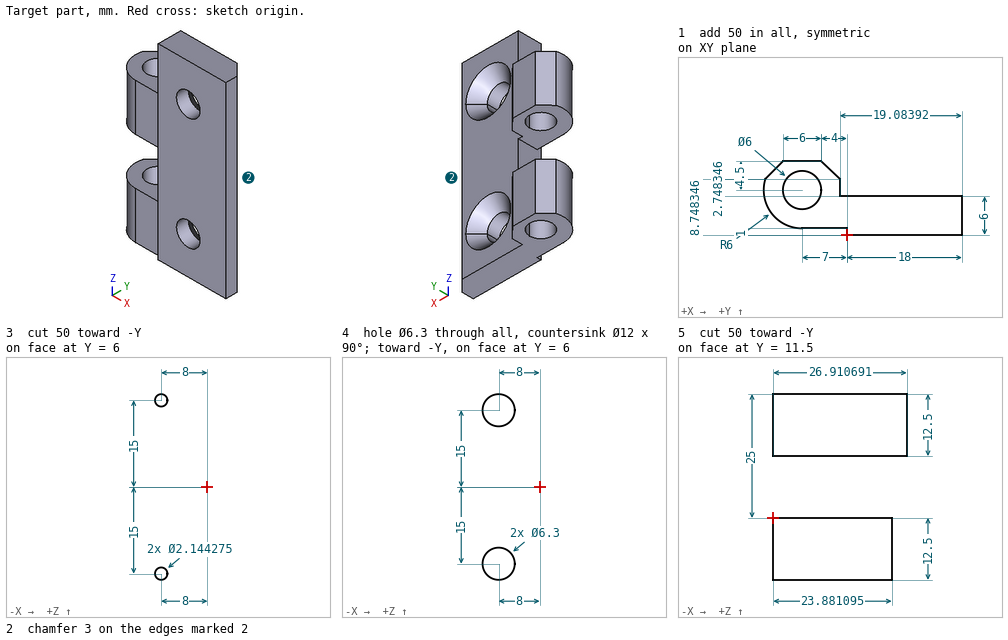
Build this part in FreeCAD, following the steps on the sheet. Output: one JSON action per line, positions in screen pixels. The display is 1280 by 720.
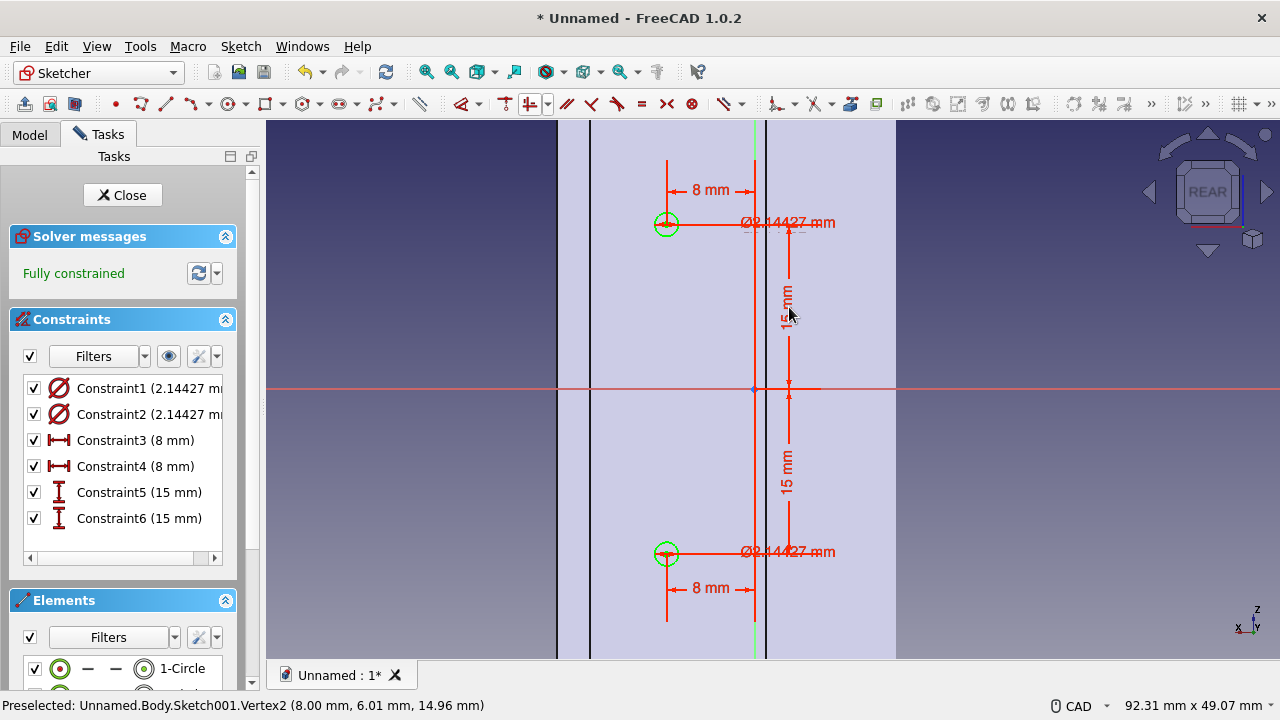
{"action": "left_click", "coordinate": [123, 195]}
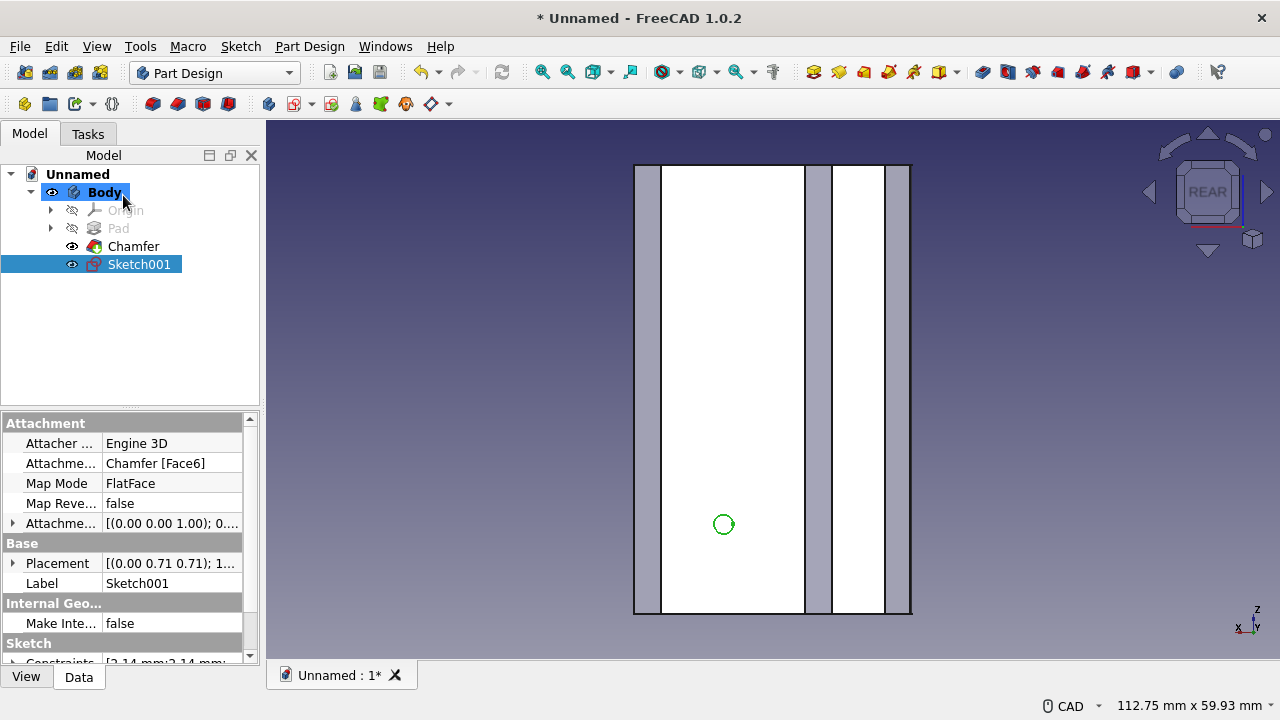
{"action": "left_click", "coordinate": [983, 72]}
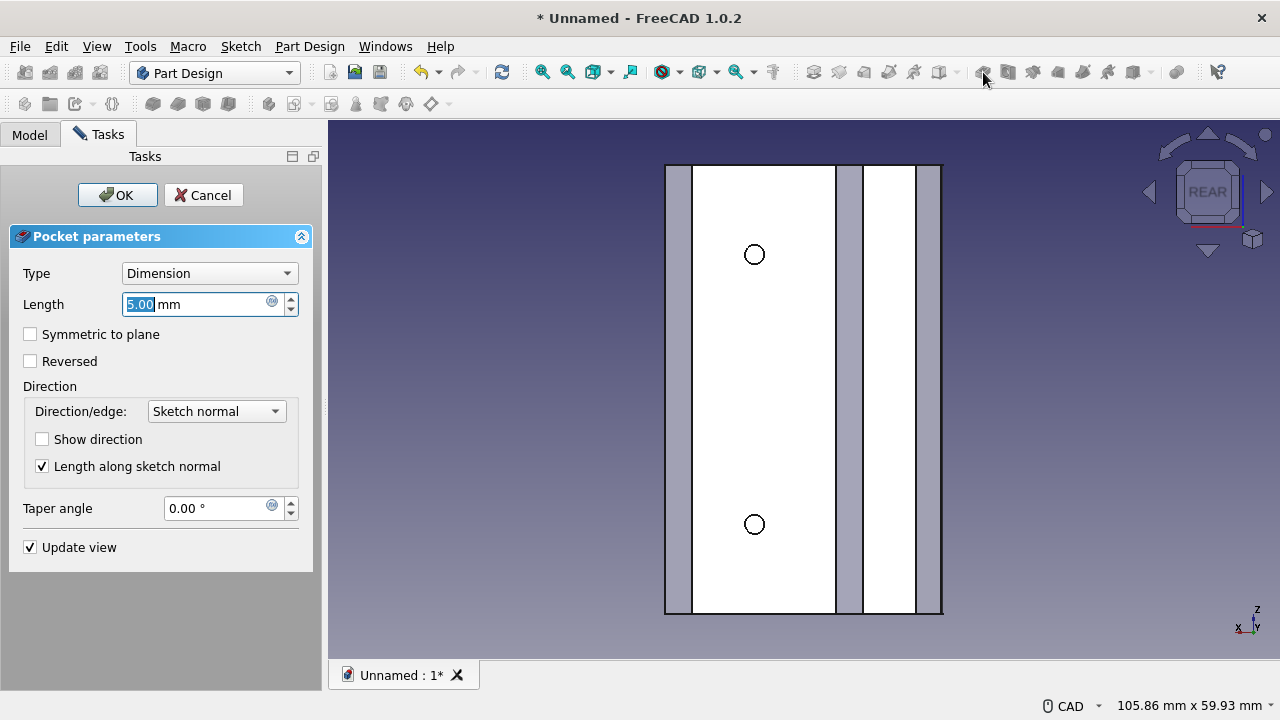
{"action": "type", "text": "50"}
{"action": "key", "text": "Tab"}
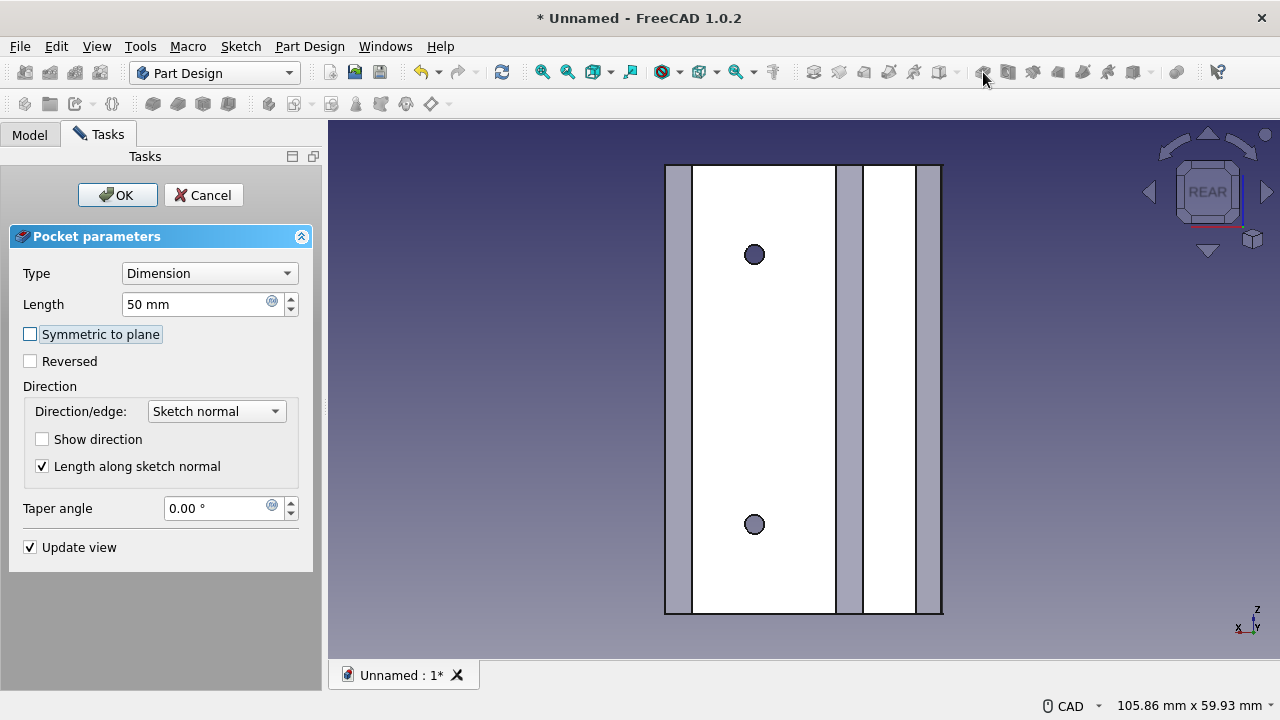
{"action": "left_click", "coordinate": [118, 195]}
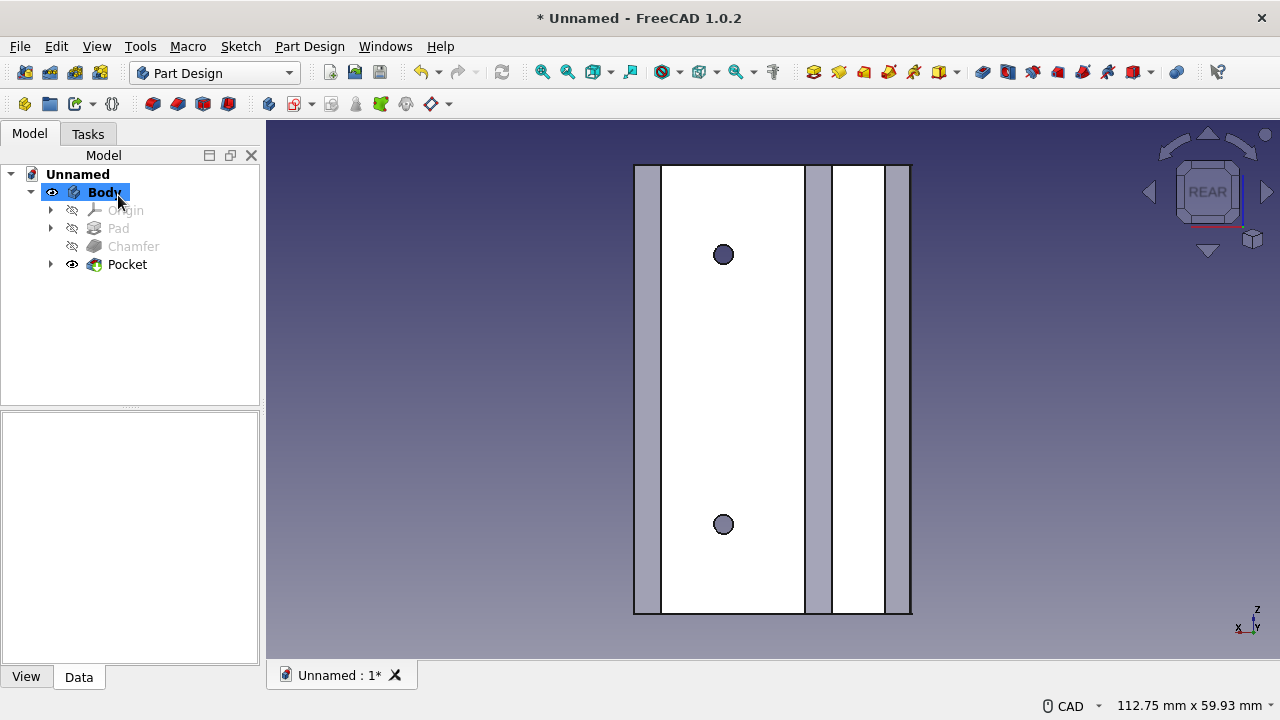
{"action": "left_click", "coordinate": [733, 388]}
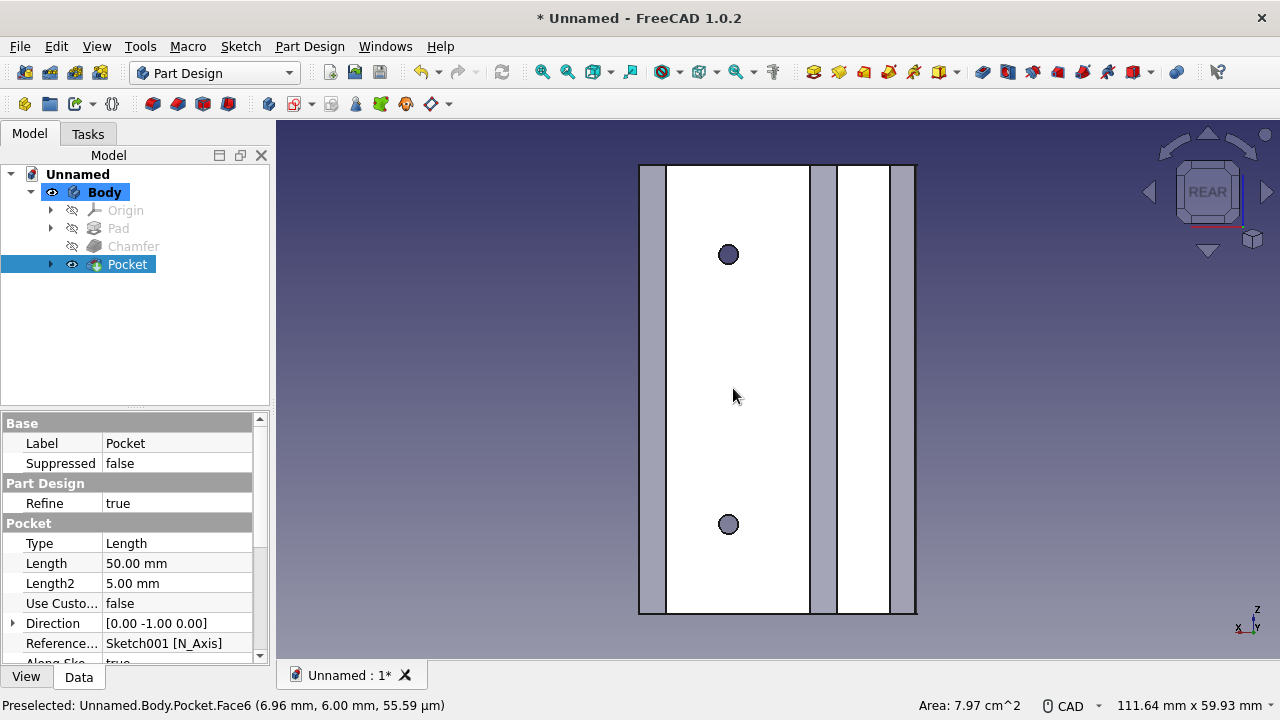
{"action": "left_click", "coordinate": [294, 104]}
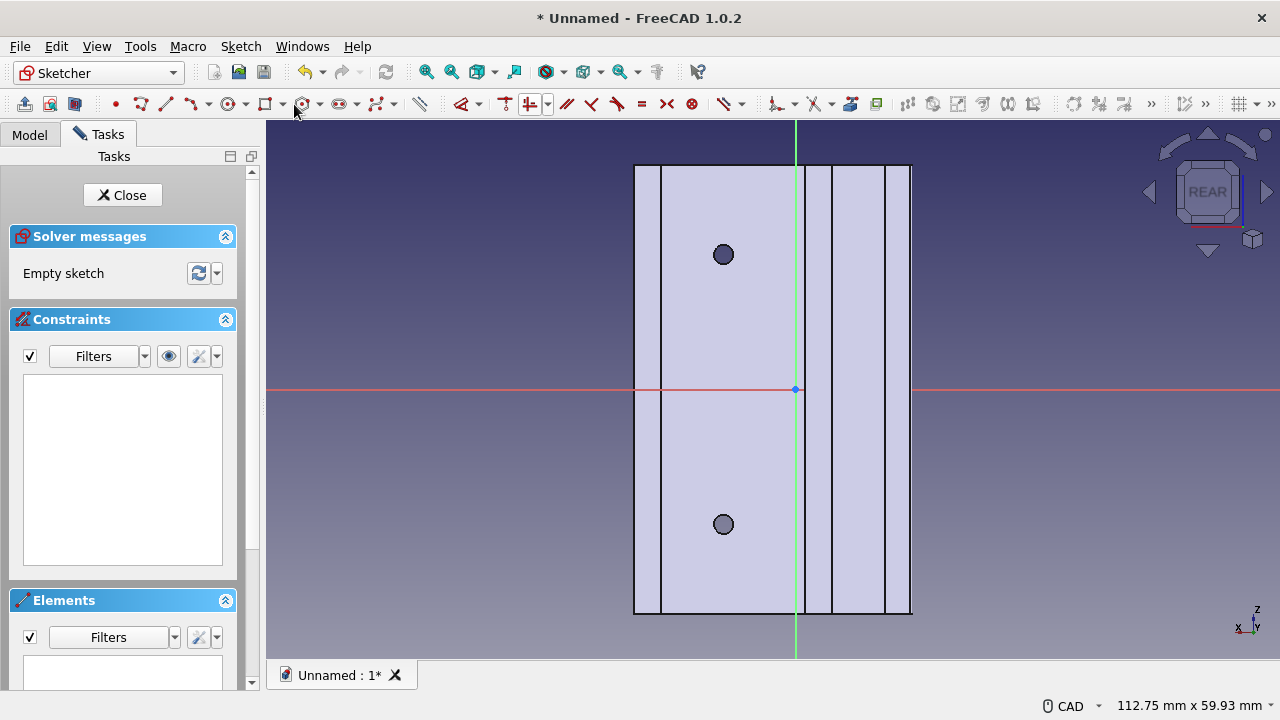
{"action": "left_click", "coordinate": [228, 104]}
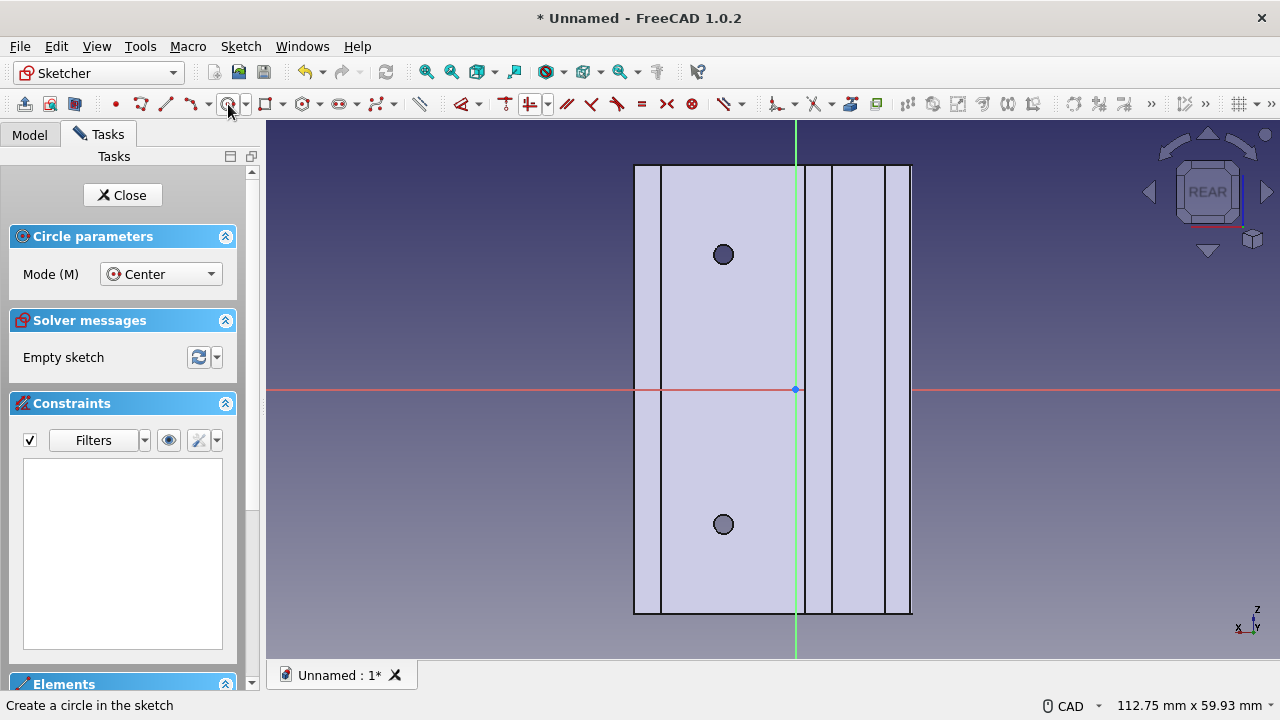
{"action": "left_click", "coordinate": [724, 524]}
{"action": "mouse_move", "coordinate": [744, 504]}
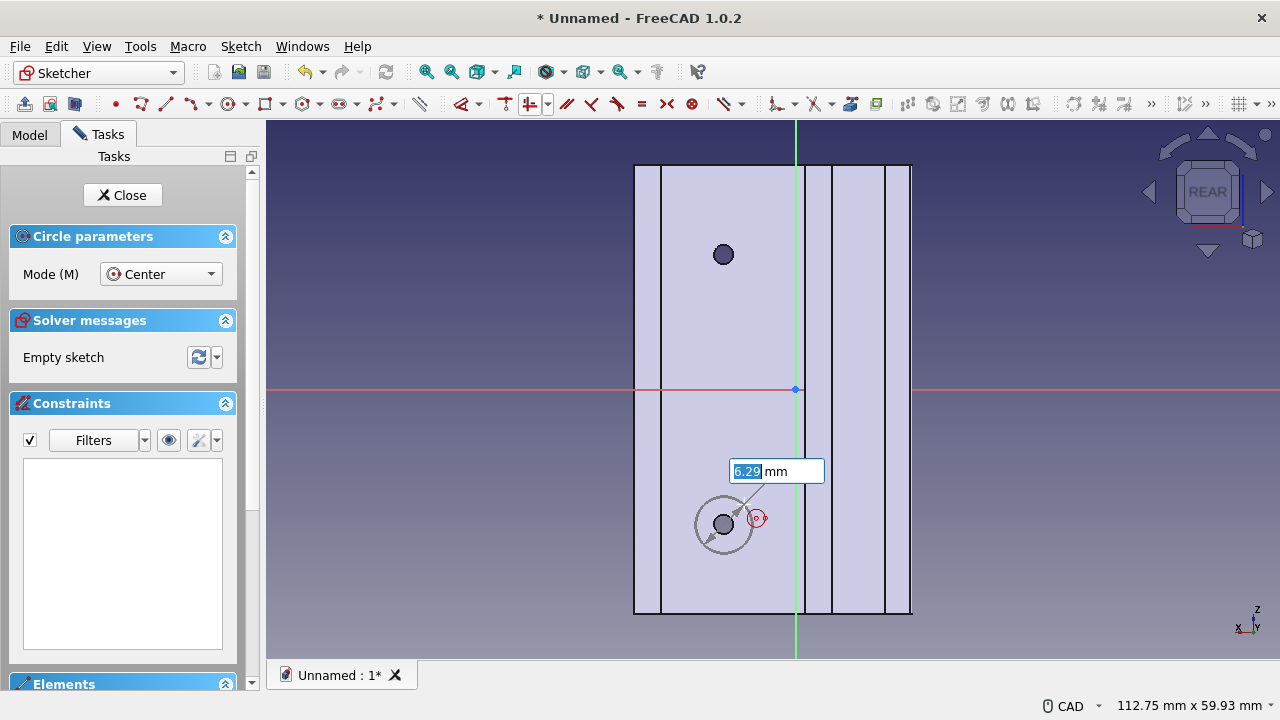
{"action": "type", "text": "6.3"}
{"action": "key", "text": "Return"}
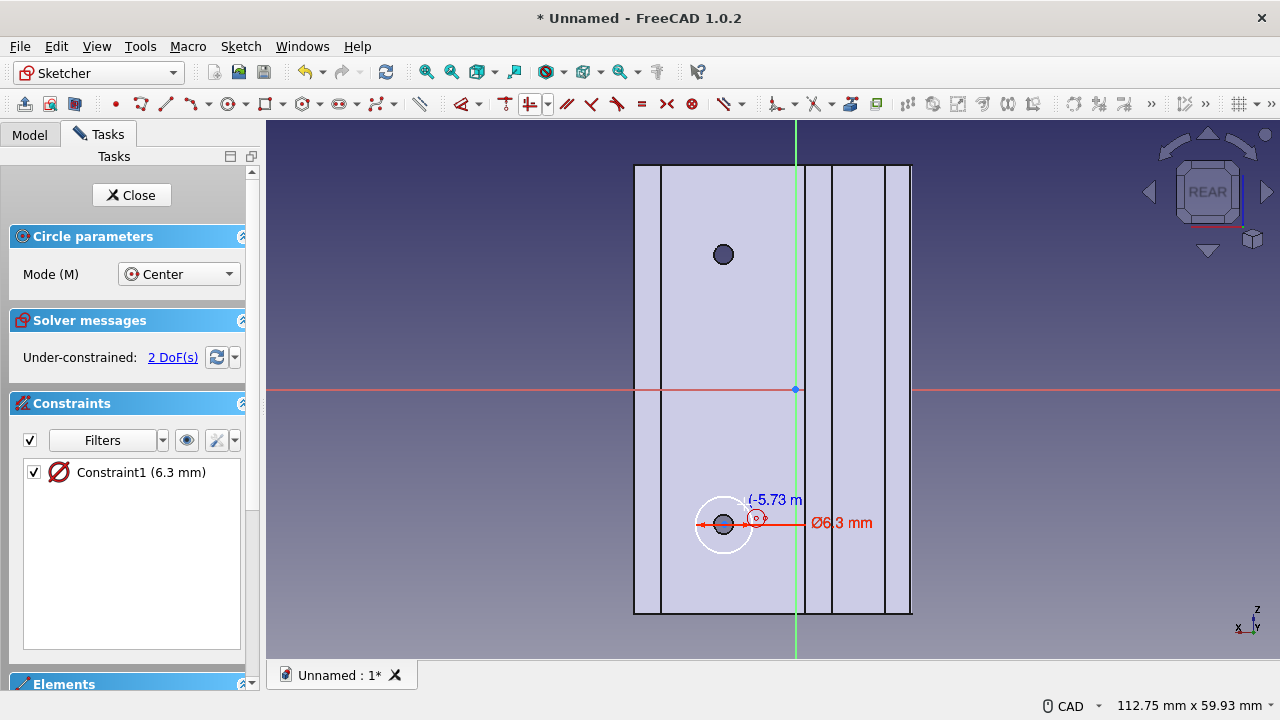
{"action": "left_click", "coordinate": [724, 255]}
{"action": "mouse_move", "coordinate": [744, 235]}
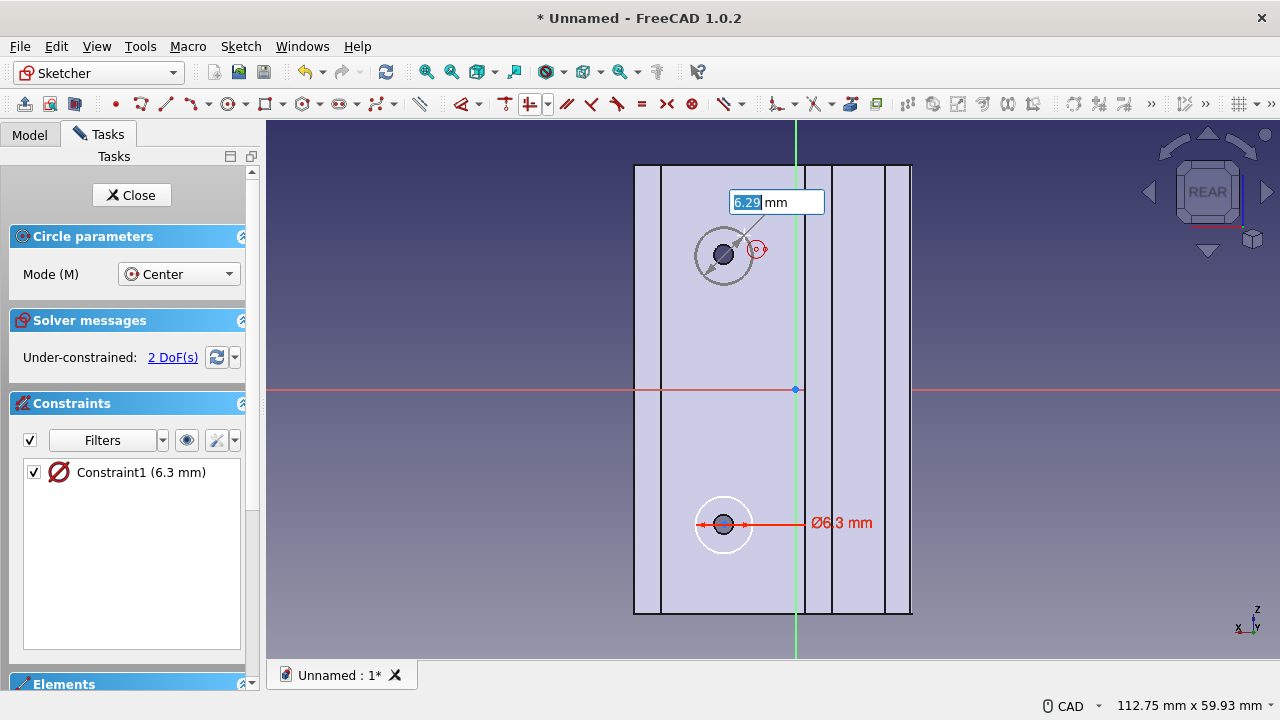
{"action": "type", "text": "6.3"}
{"action": "key", "text": "Return"}
{"action": "key", "text": "Escape"}